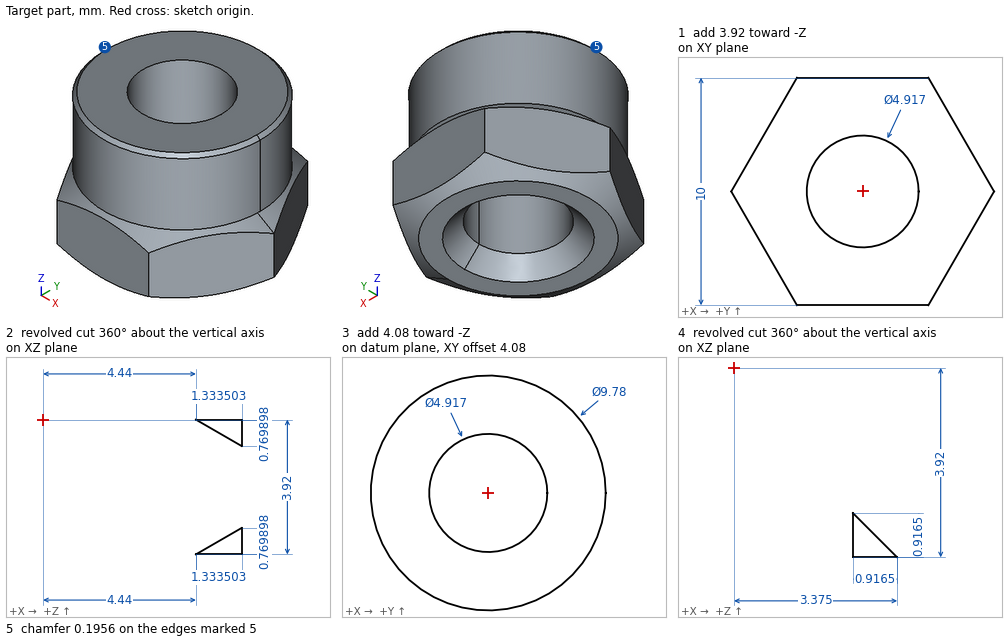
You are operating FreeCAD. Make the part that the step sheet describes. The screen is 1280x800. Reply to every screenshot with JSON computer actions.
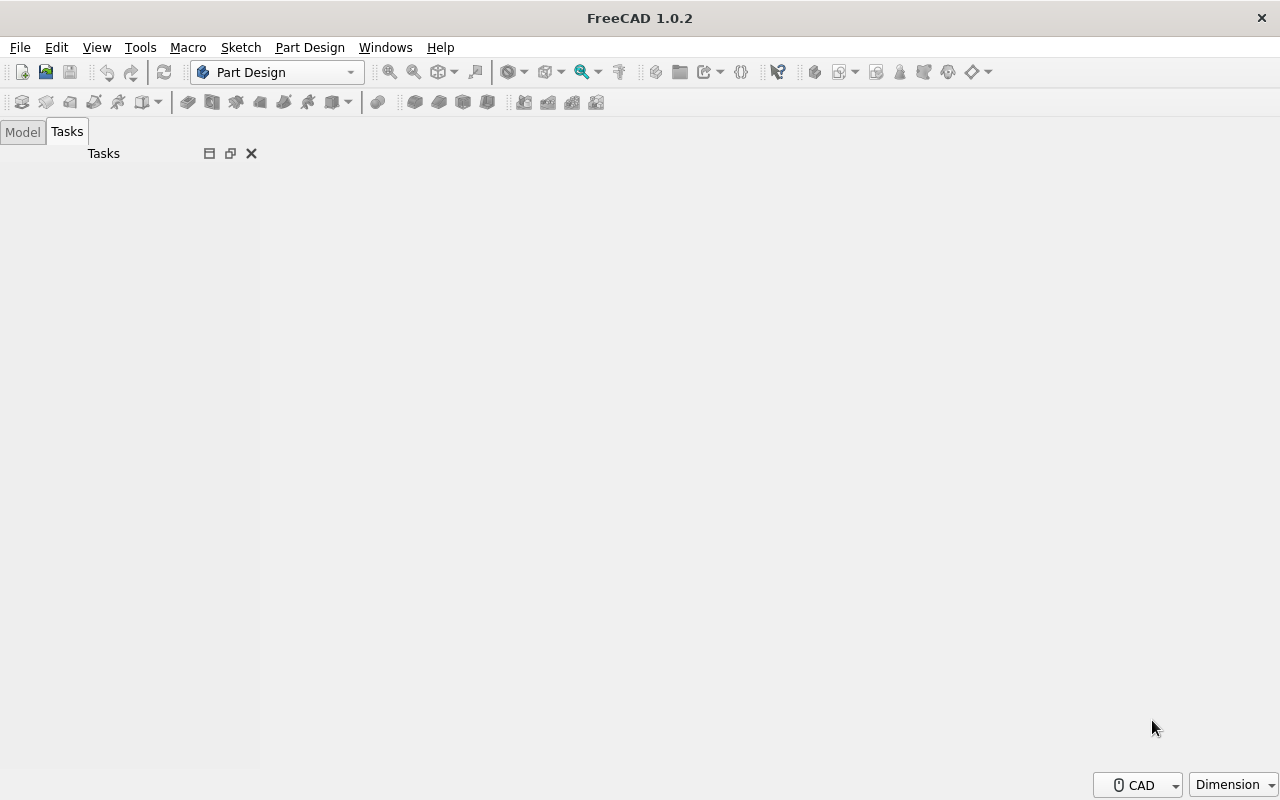
{"action": "key", "text": "ctrl+n"}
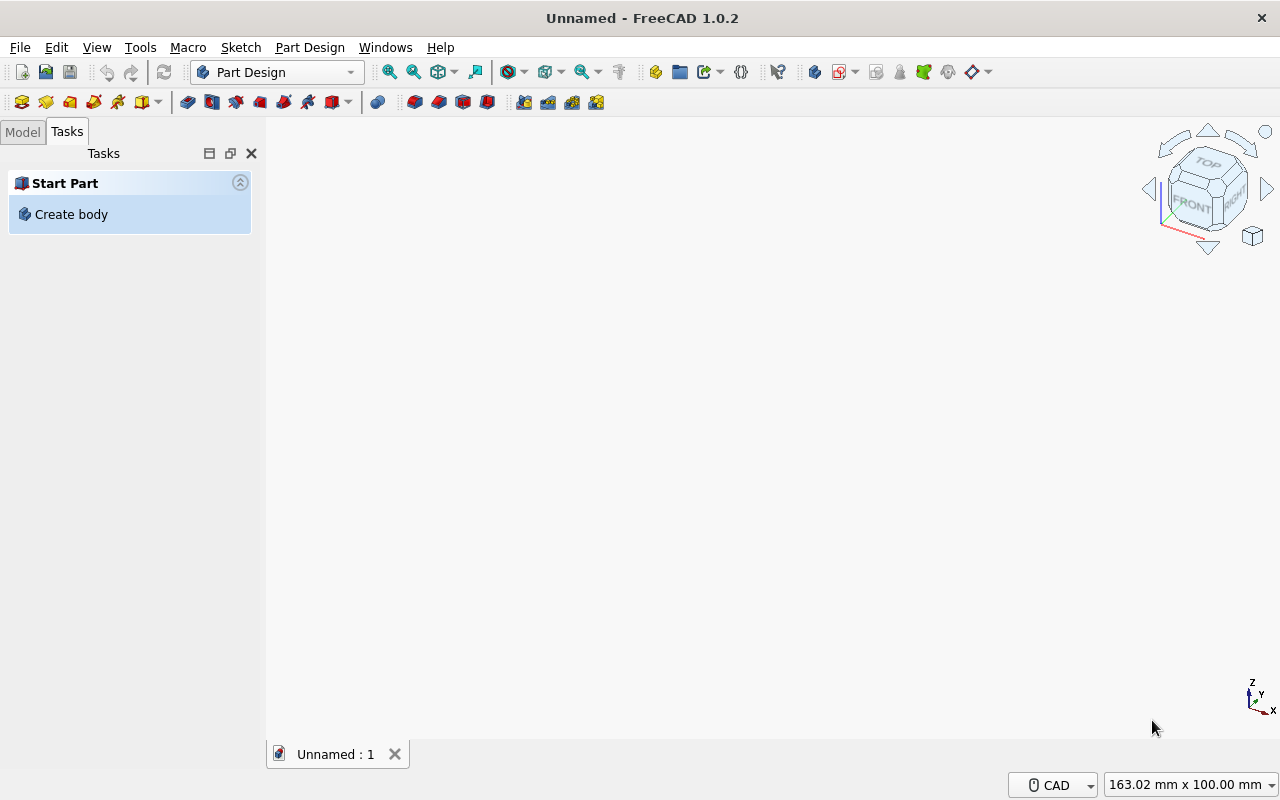
{"action": "left_click", "coordinate": [840, 72]}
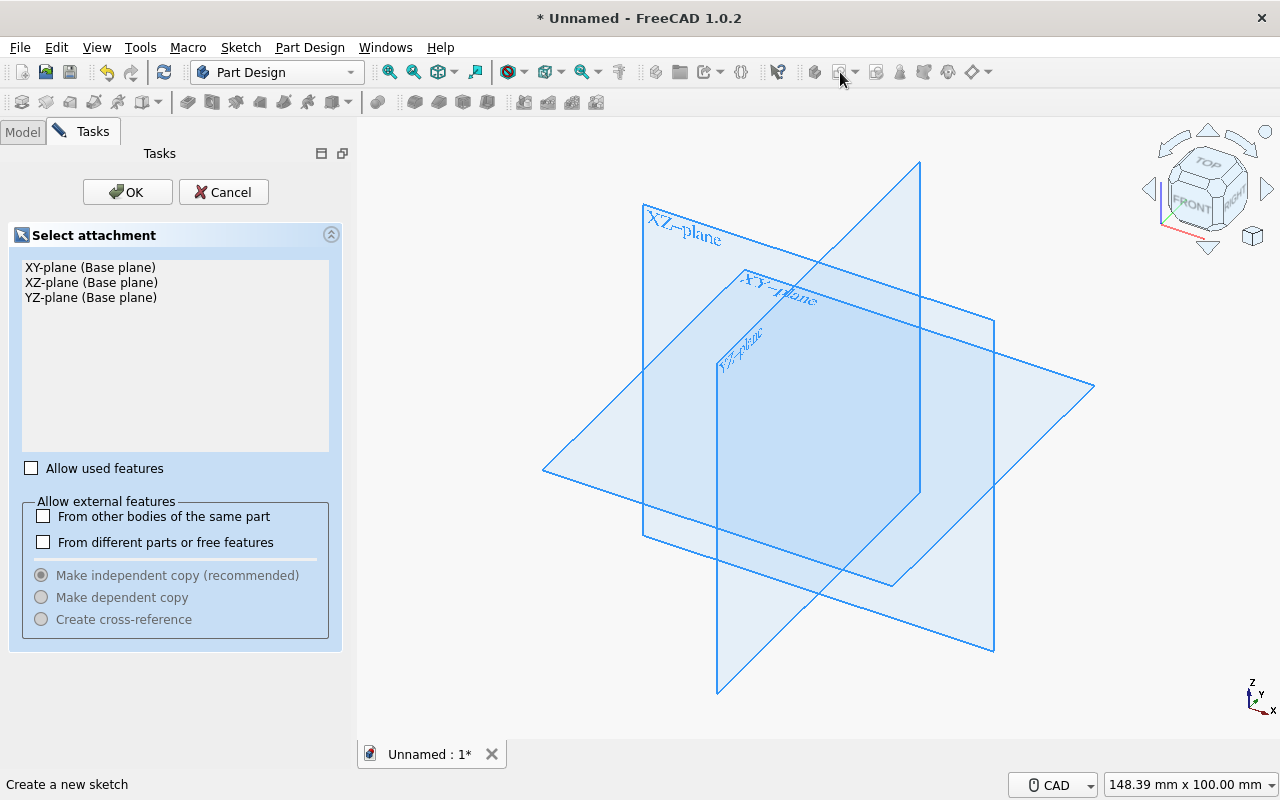
{"action": "left_click", "coordinate": [82, 268]}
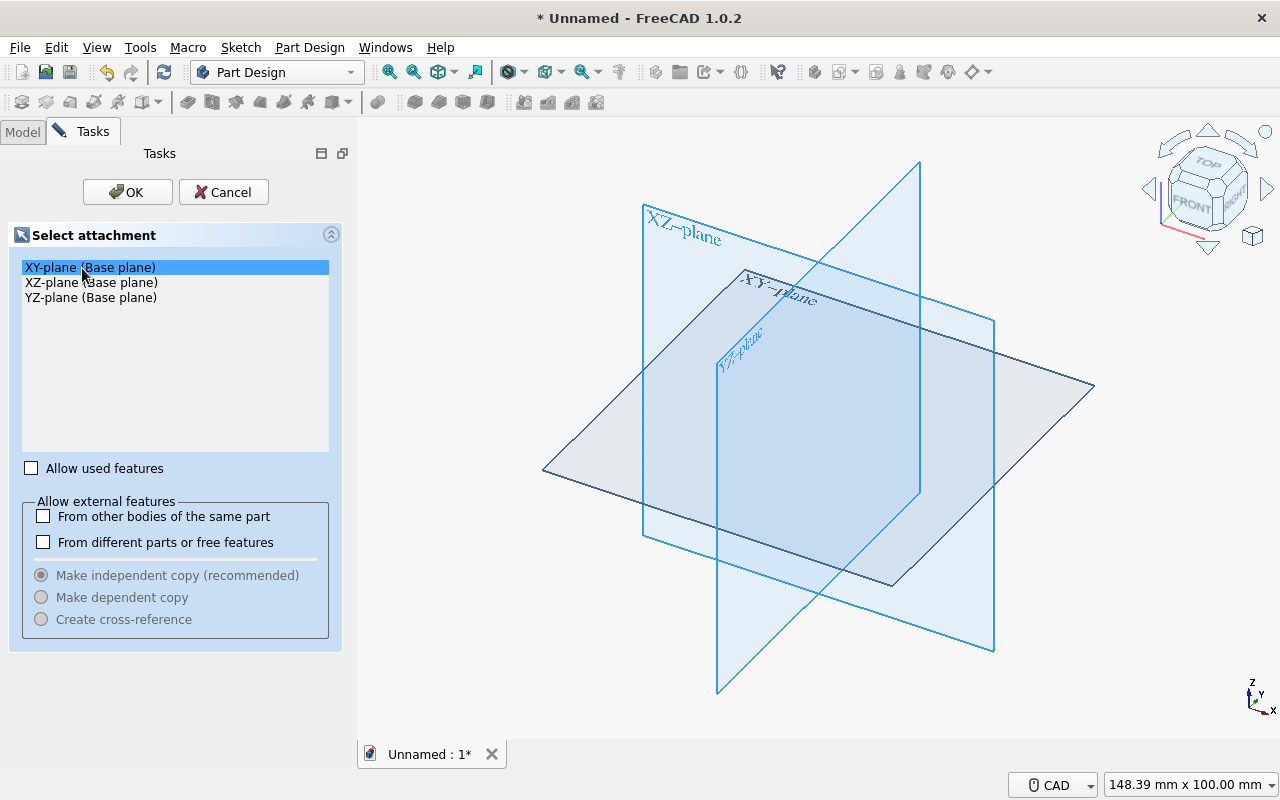
{"action": "left_click", "coordinate": [128, 192]}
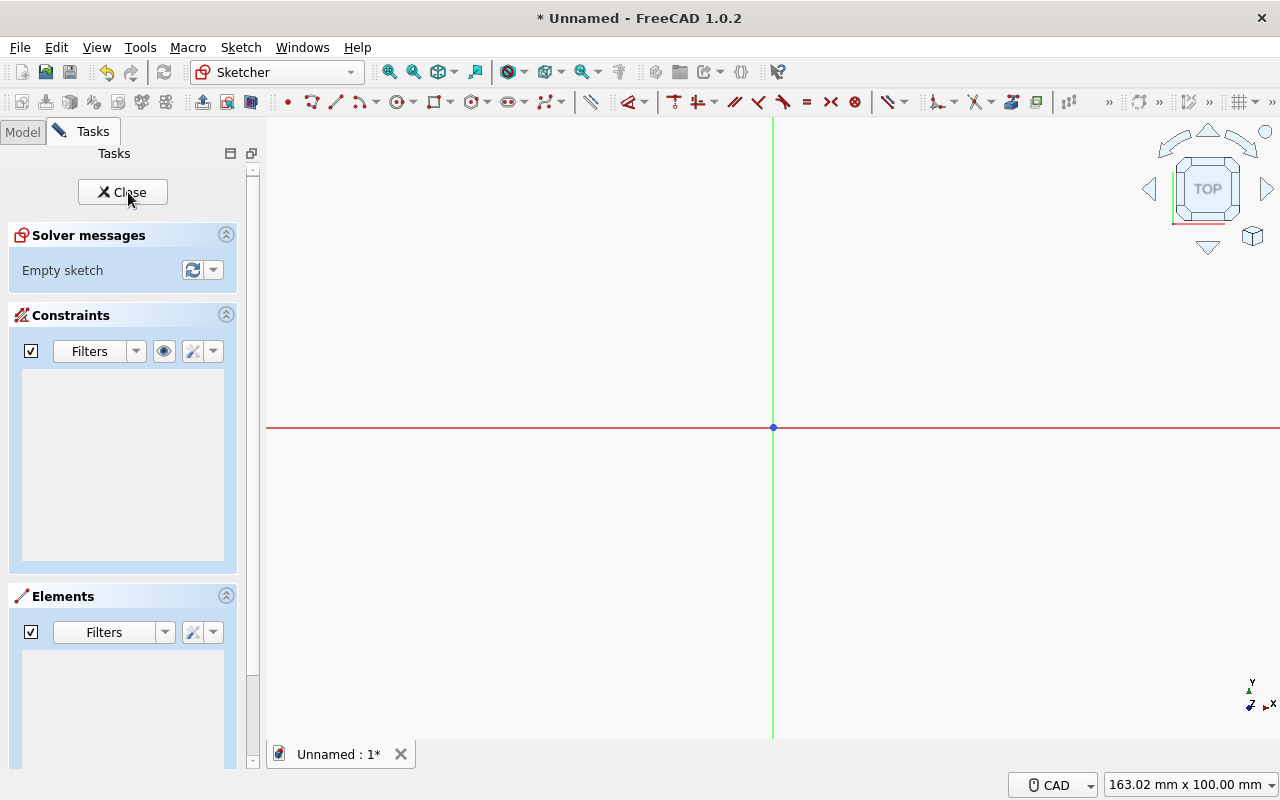
{"action": "scroll", "coordinate": [787, 428], "scroll_direction": "up", "scroll_amount": 9}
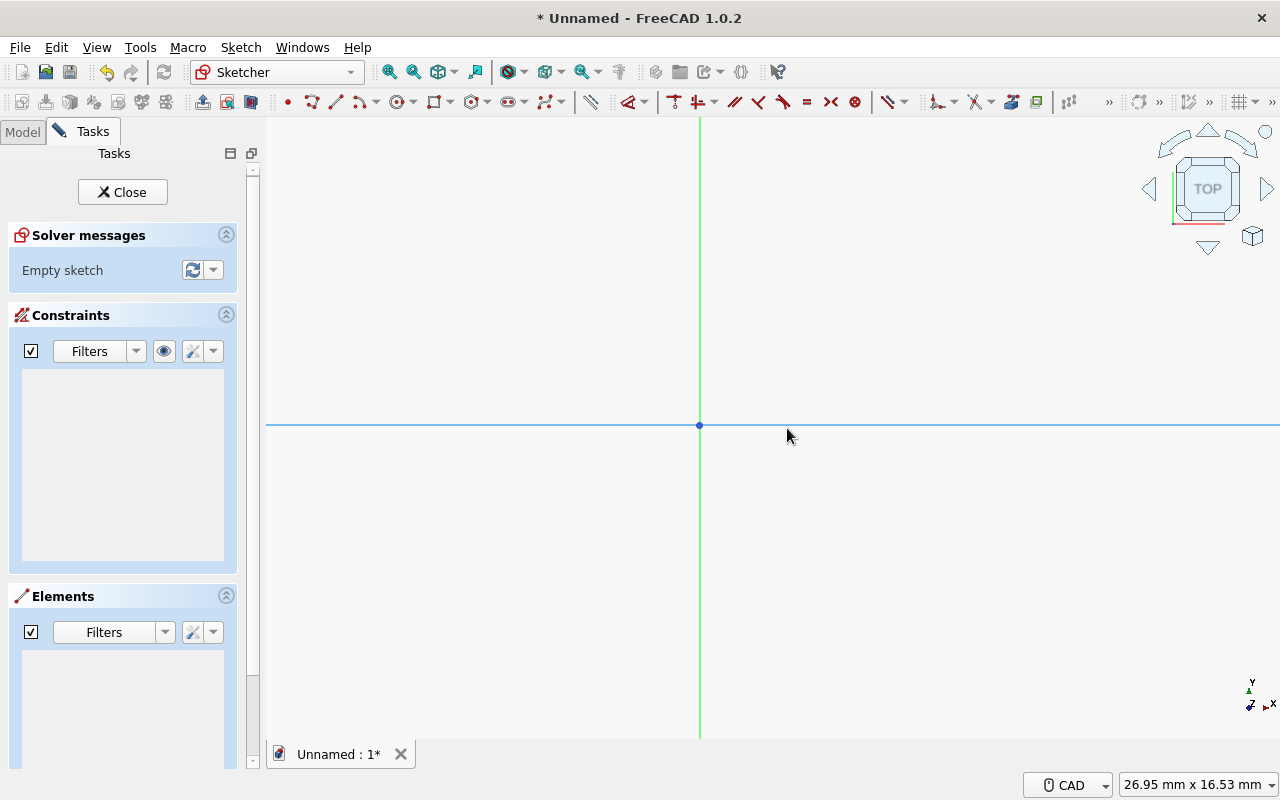
{"action": "key", "text": "g p 6"}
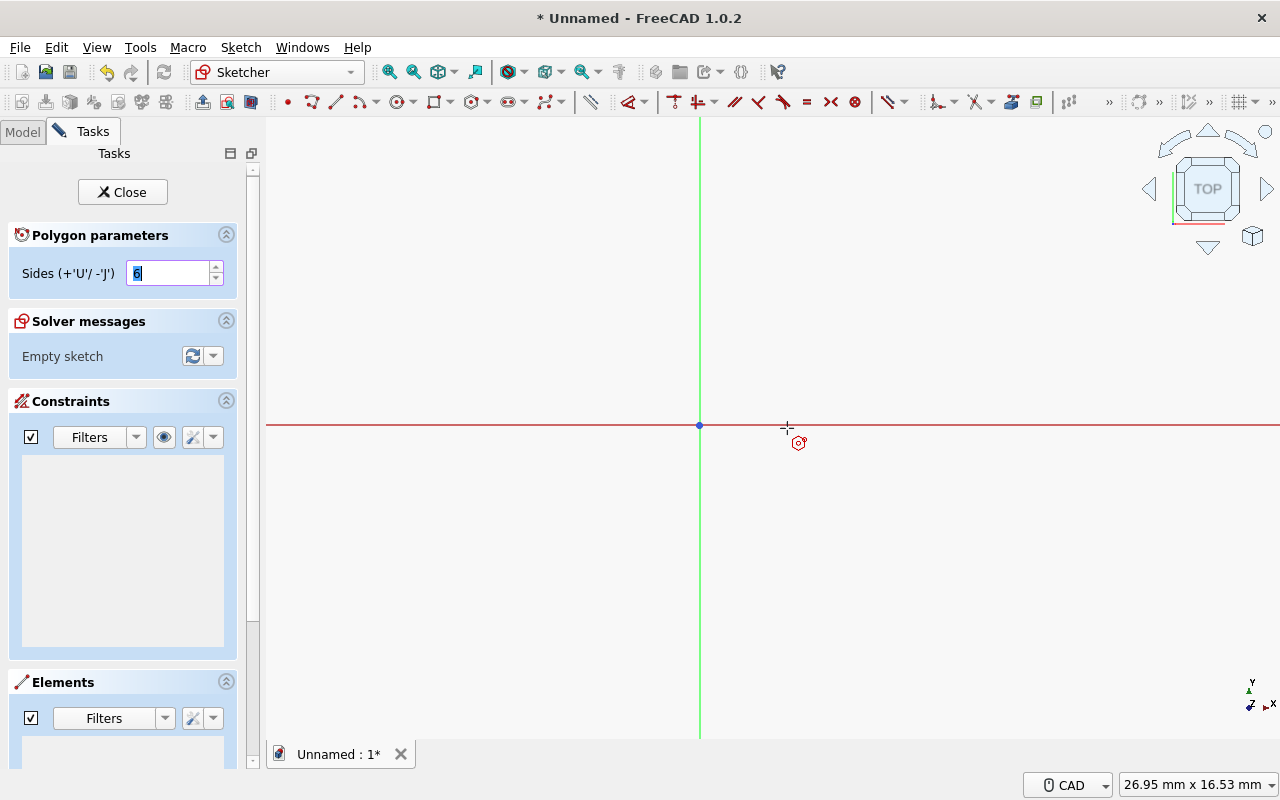
{"action": "left_click", "coordinate": [700, 425]}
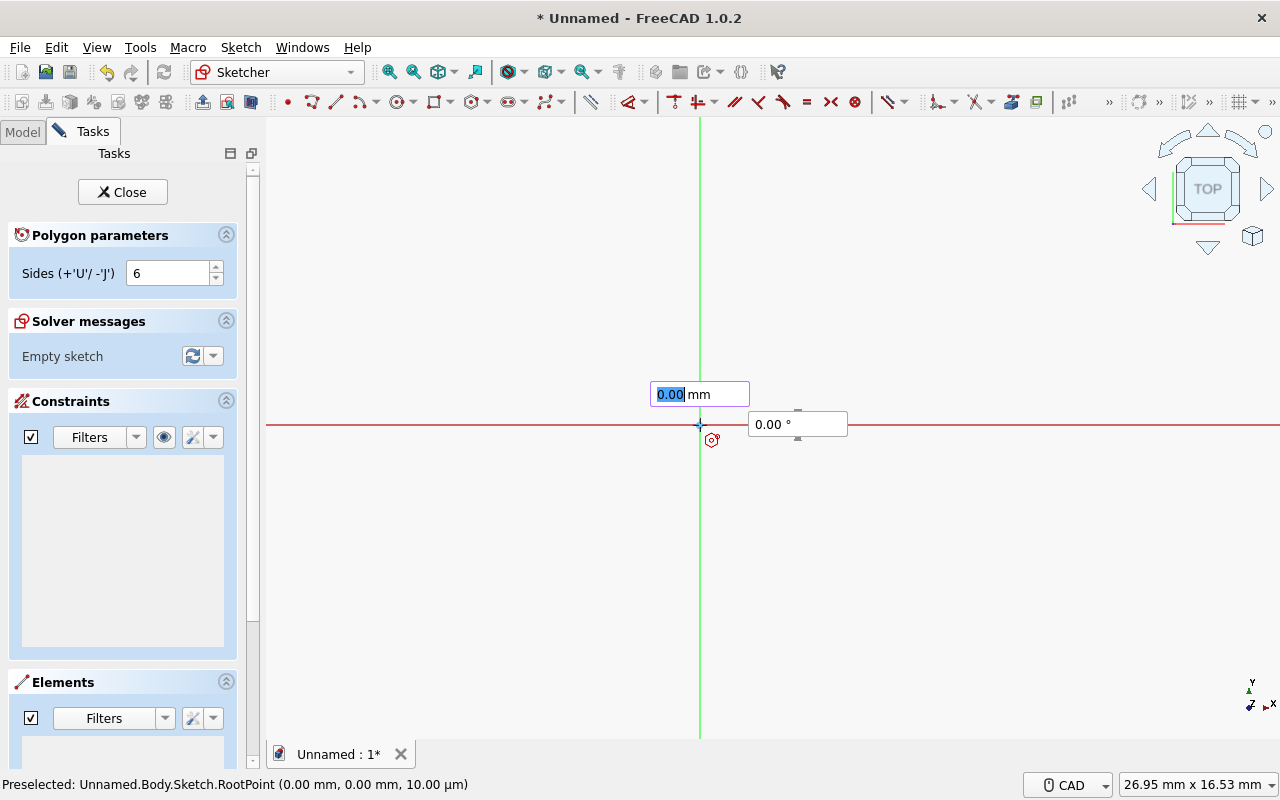
{"action": "left_click", "coordinate": [917, 425]}
{"action": "right_click", "coordinate": [917, 425]}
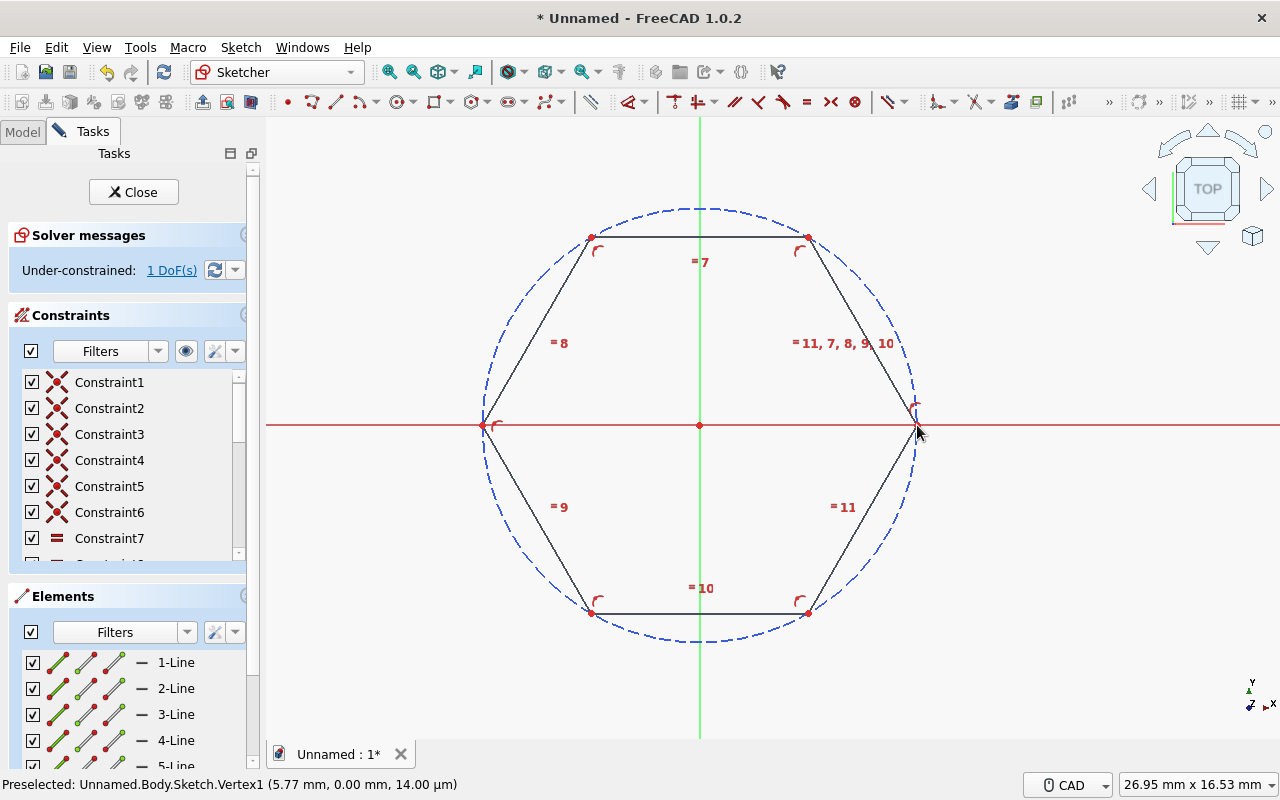
{"action": "key", "text": "g c"}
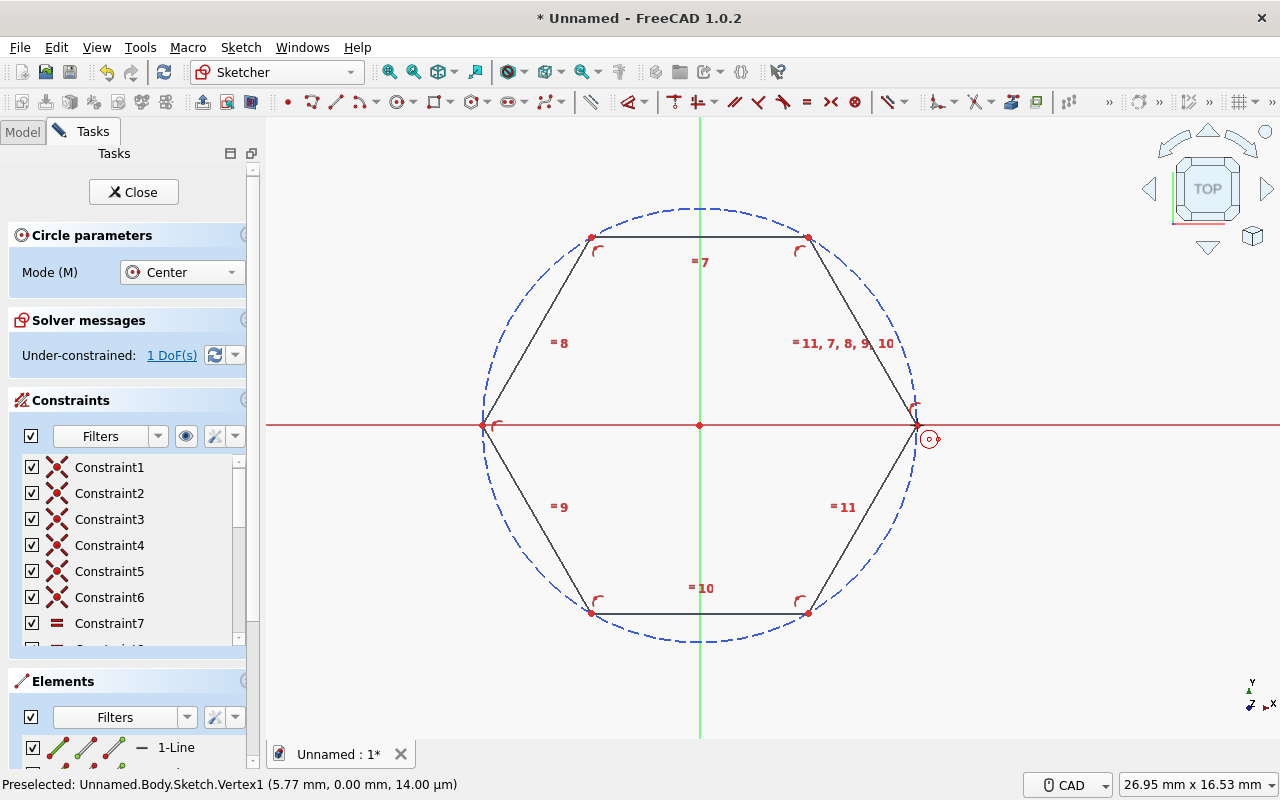
{"action": "left_click", "coordinate": [700, 425]}
{"action": "mouse_move", "coordinate": [765, 360]}